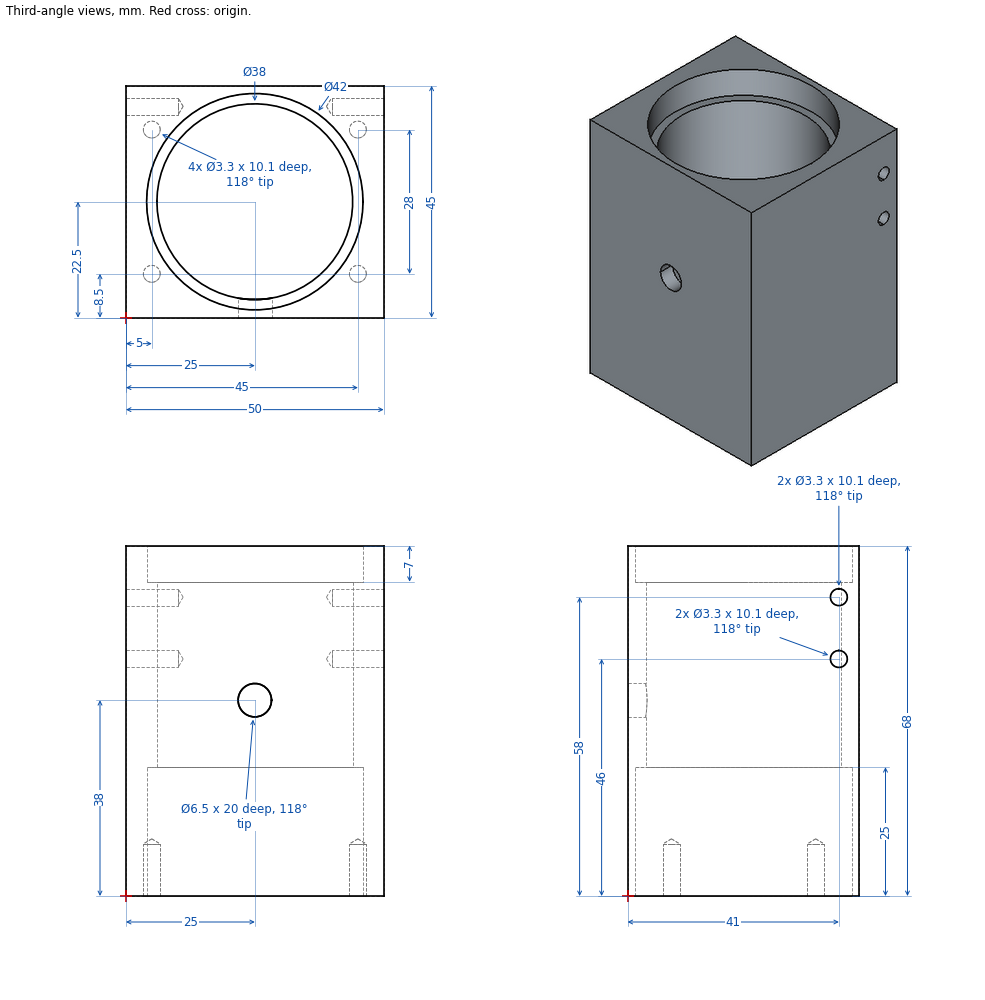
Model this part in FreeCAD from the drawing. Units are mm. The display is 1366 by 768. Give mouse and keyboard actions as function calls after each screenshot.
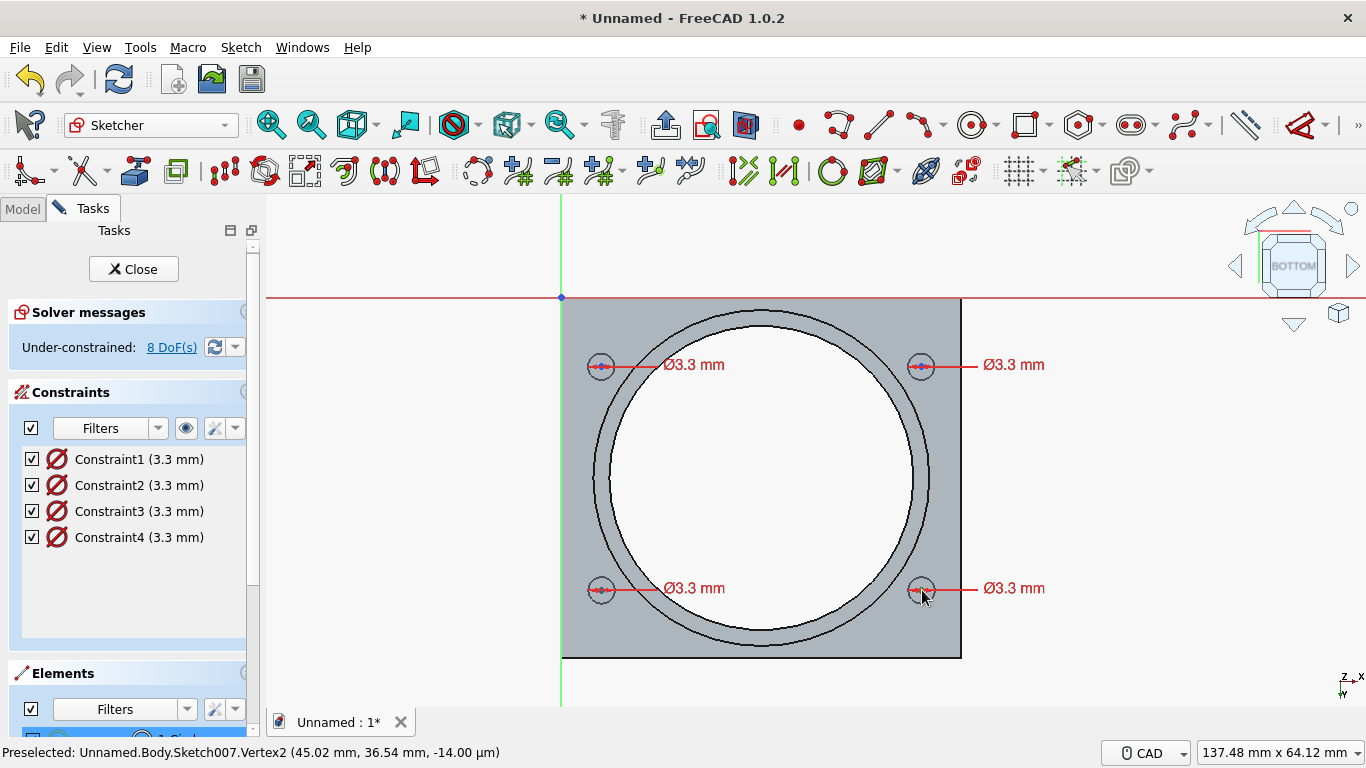
key(h)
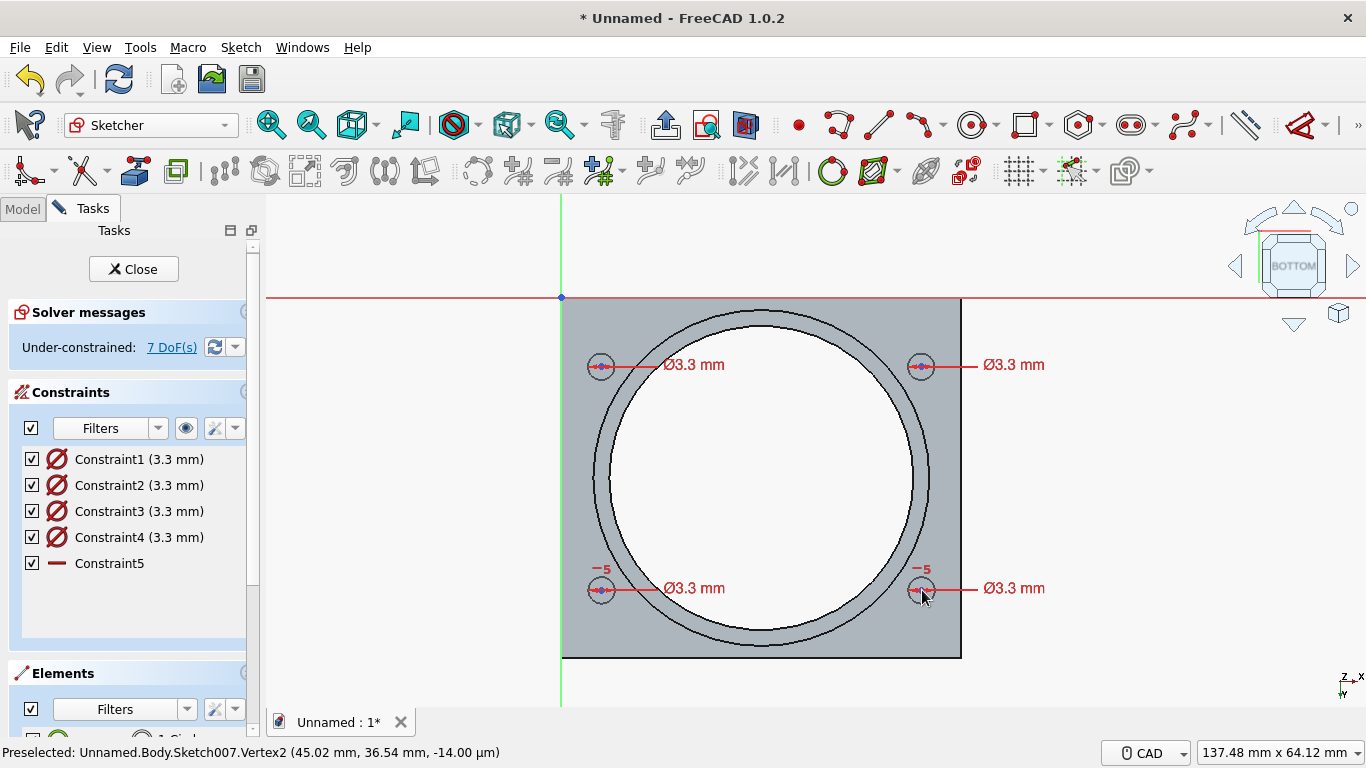
click(922, 590)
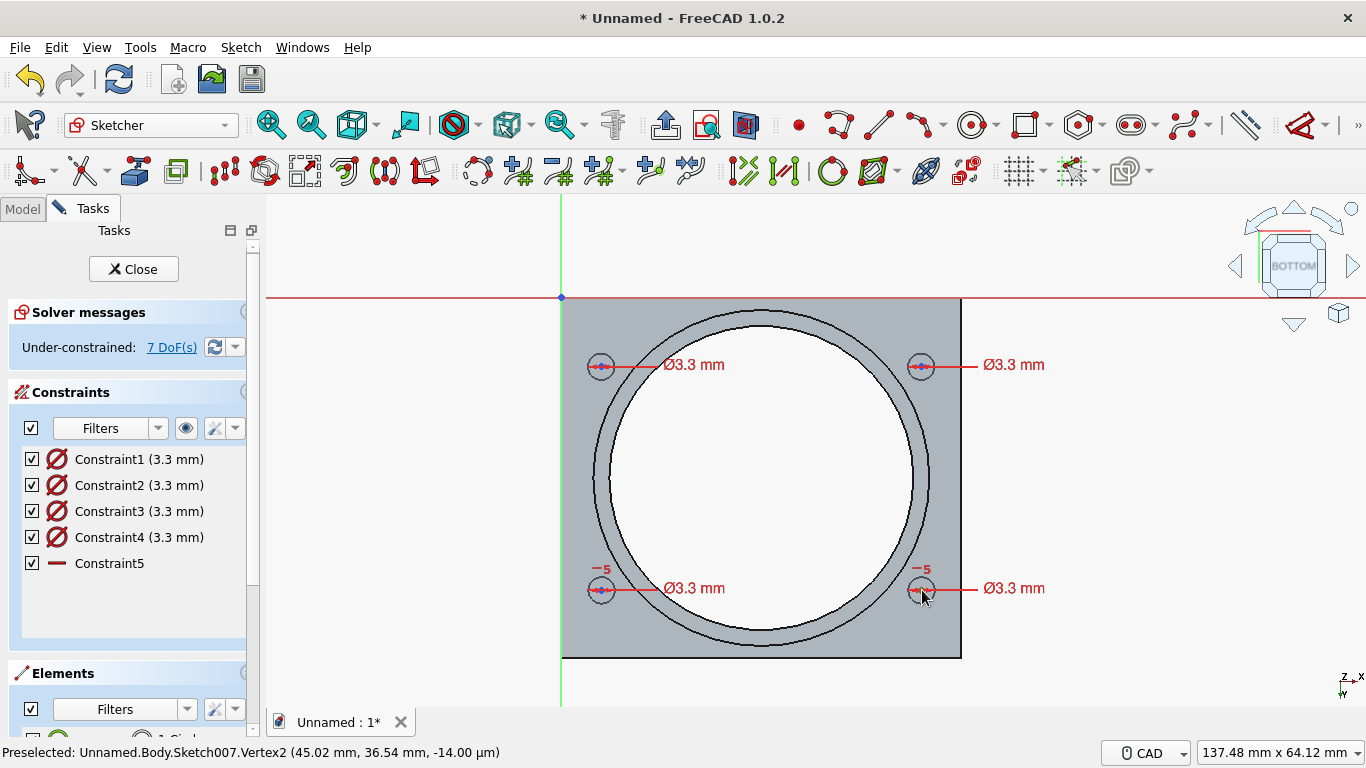
click(921, 367)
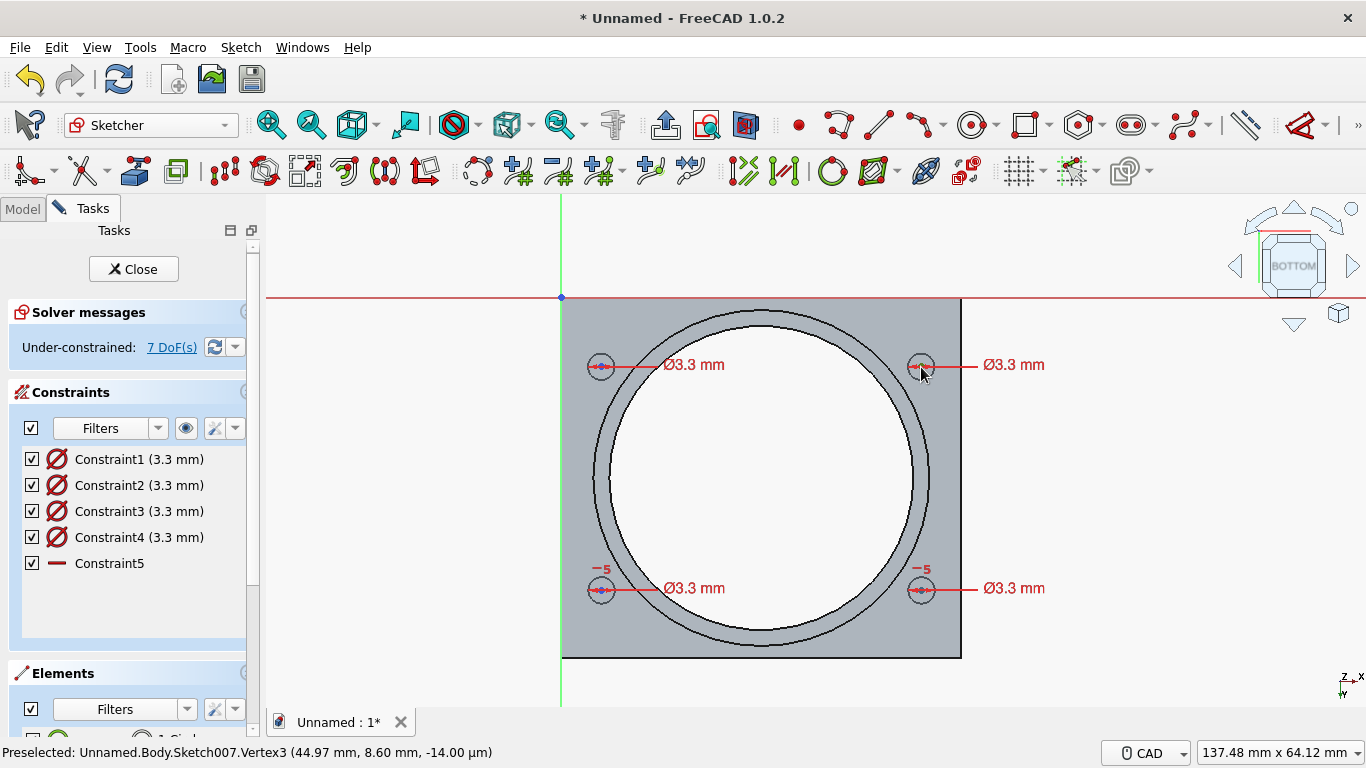
key(v)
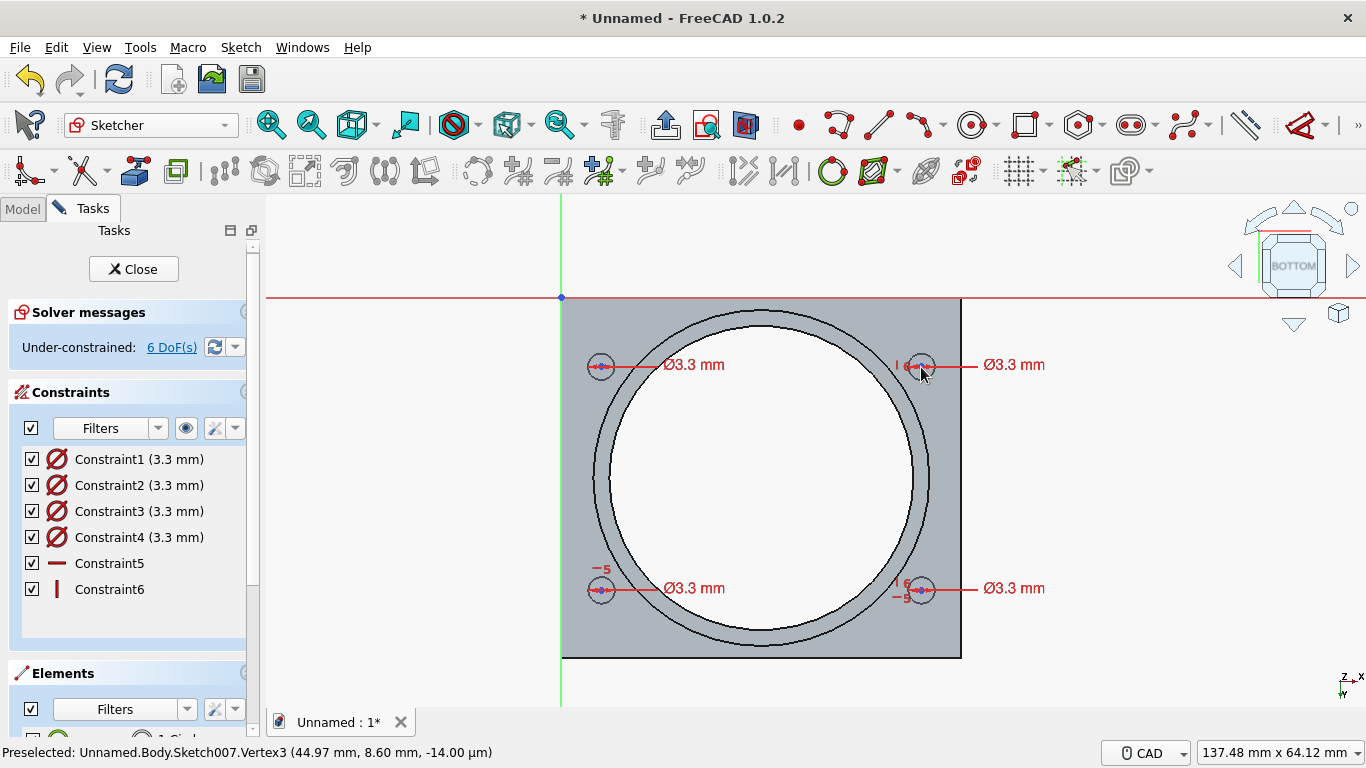
click(602, 590)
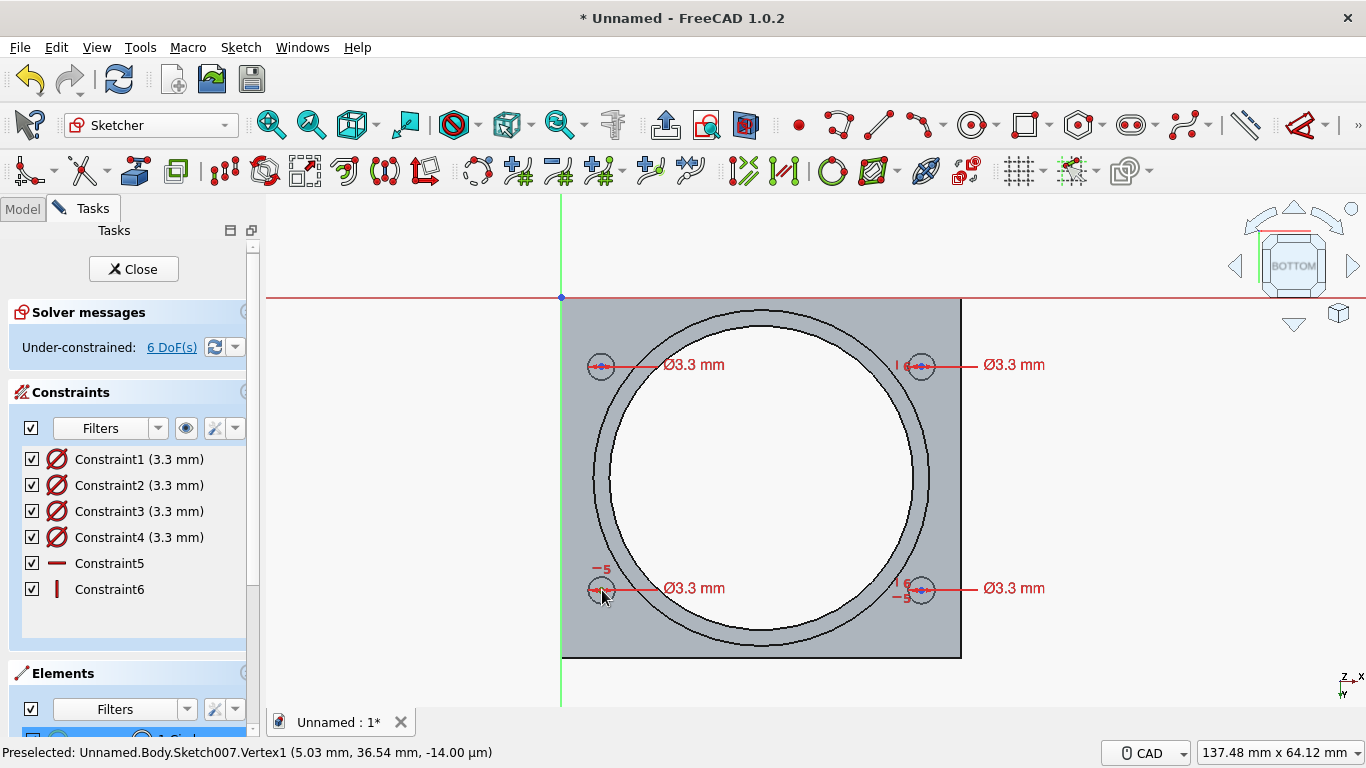
click(601, 367)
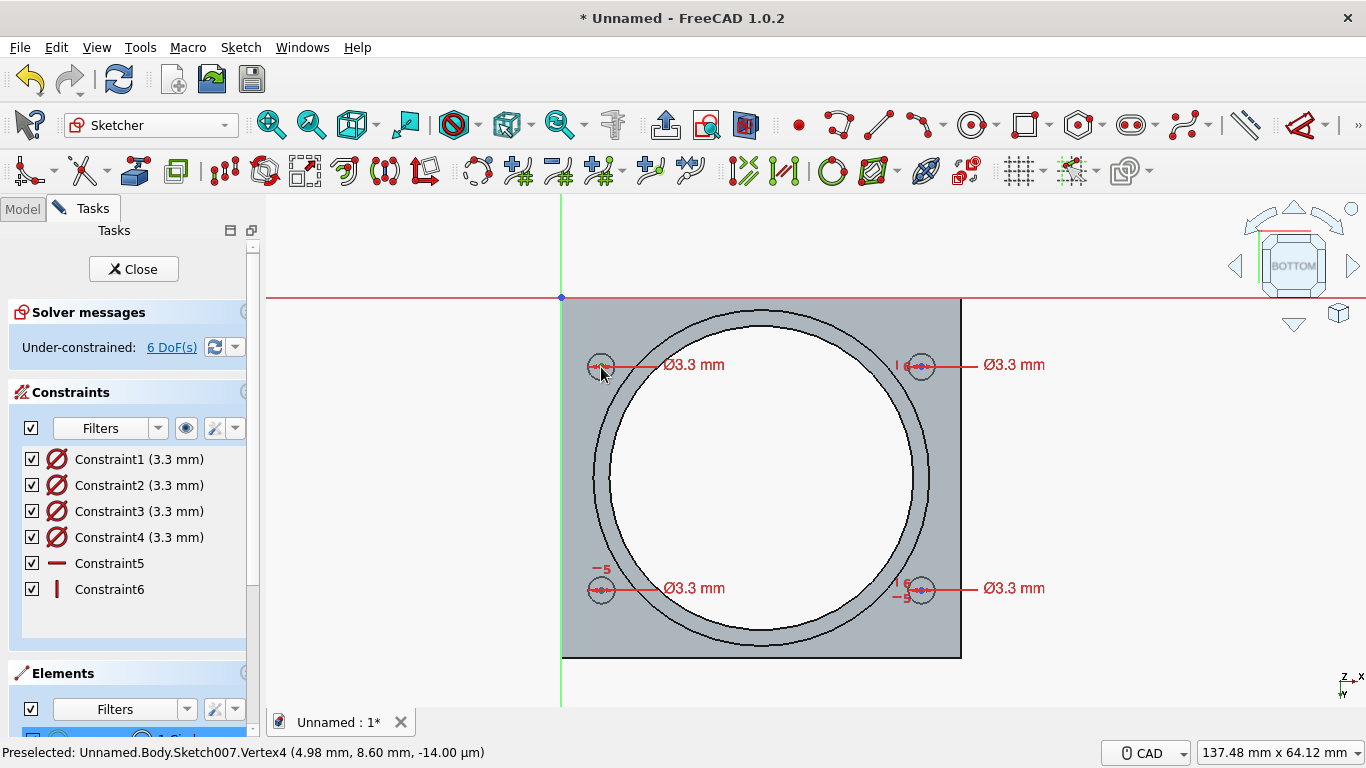
key(v)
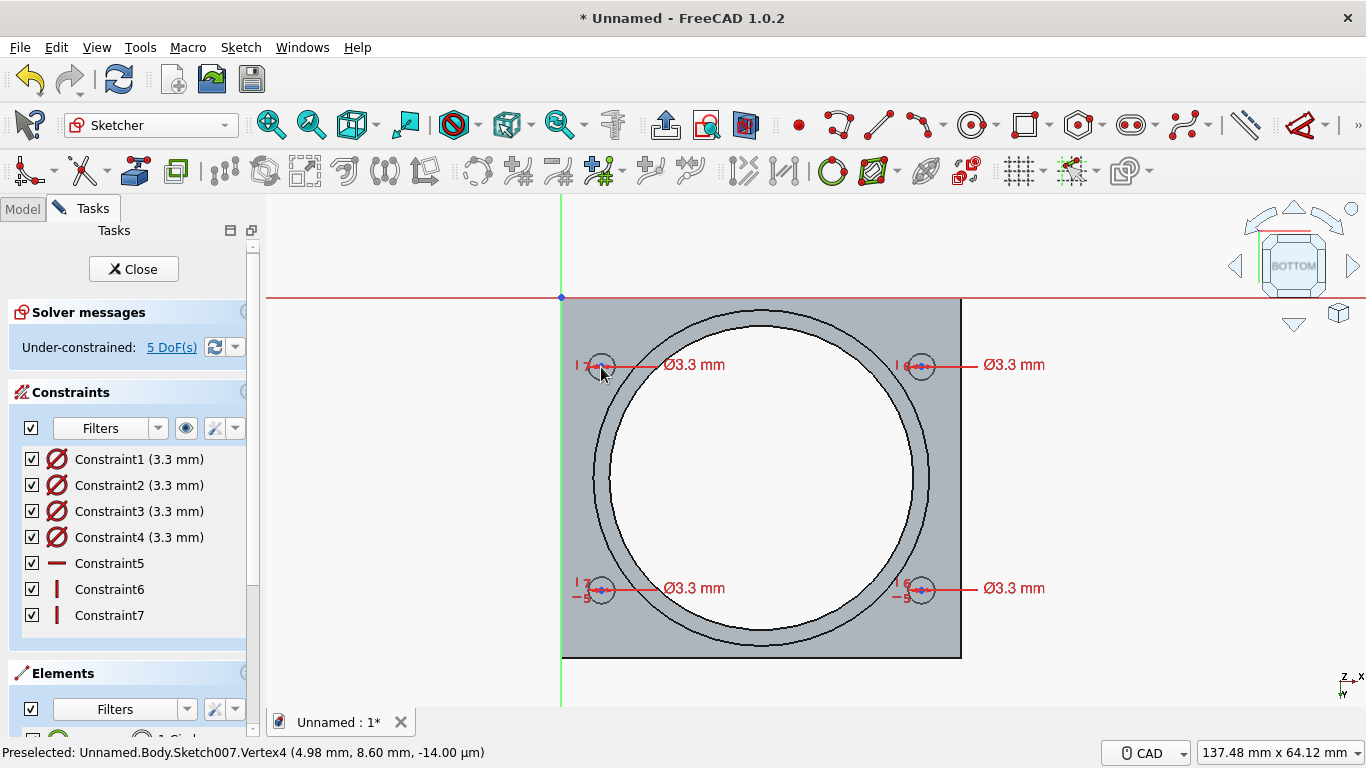
click(922, 367)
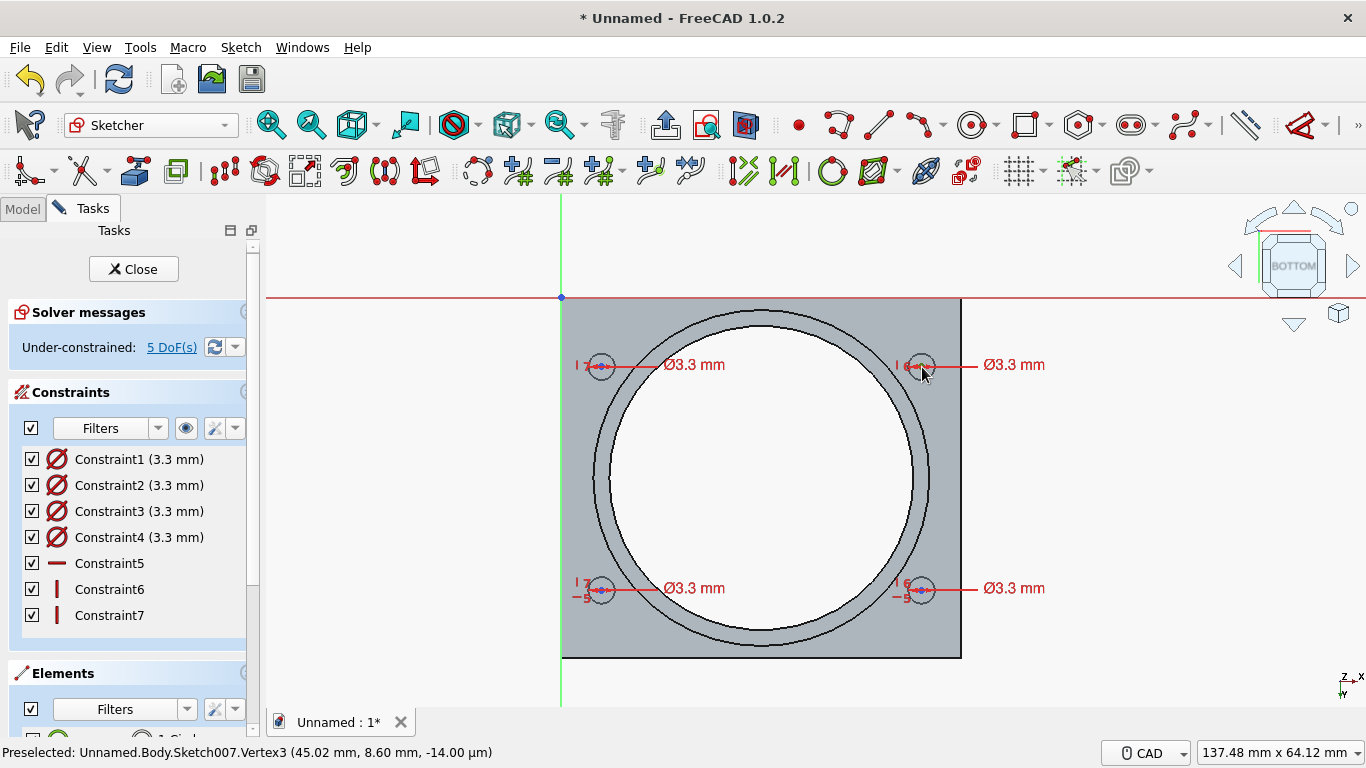
click(602, 367)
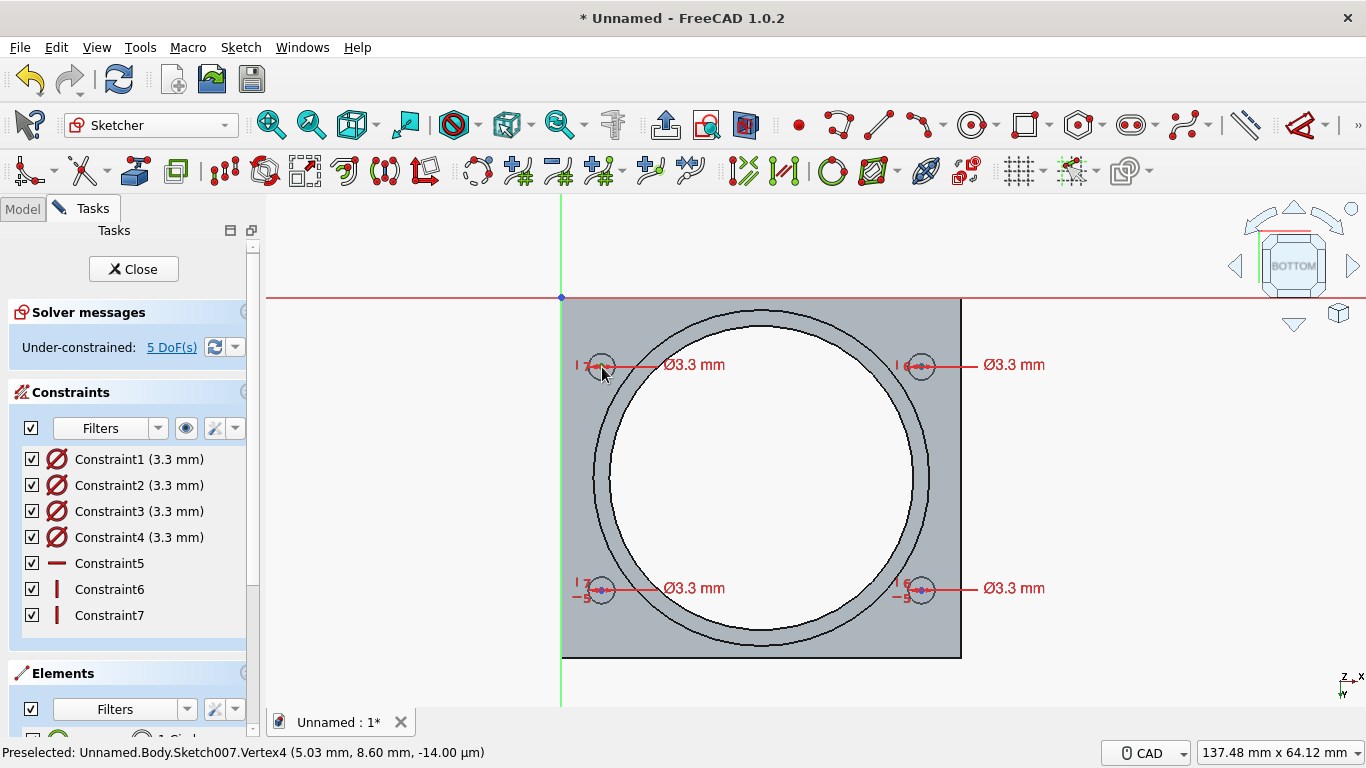
key(h)